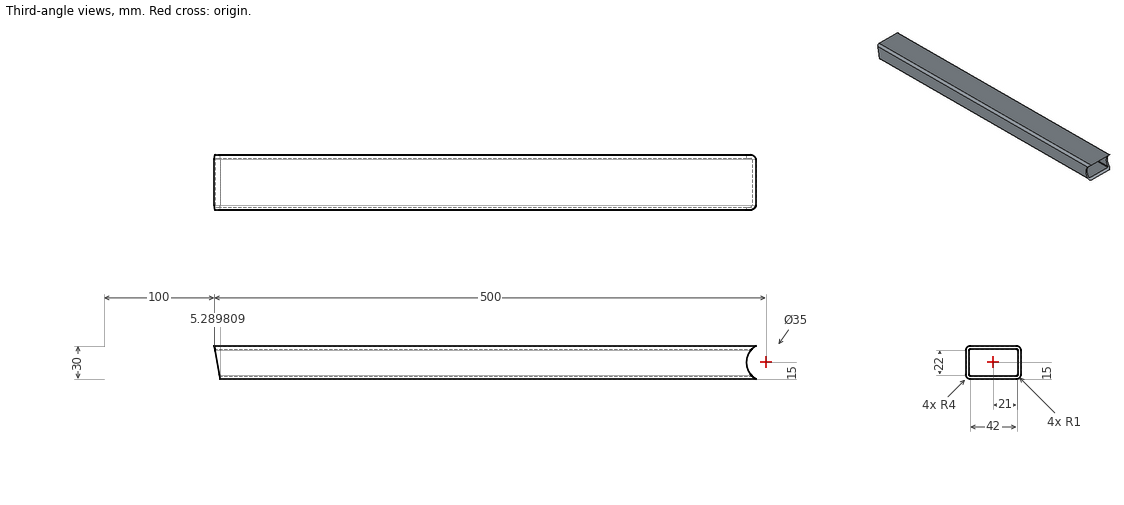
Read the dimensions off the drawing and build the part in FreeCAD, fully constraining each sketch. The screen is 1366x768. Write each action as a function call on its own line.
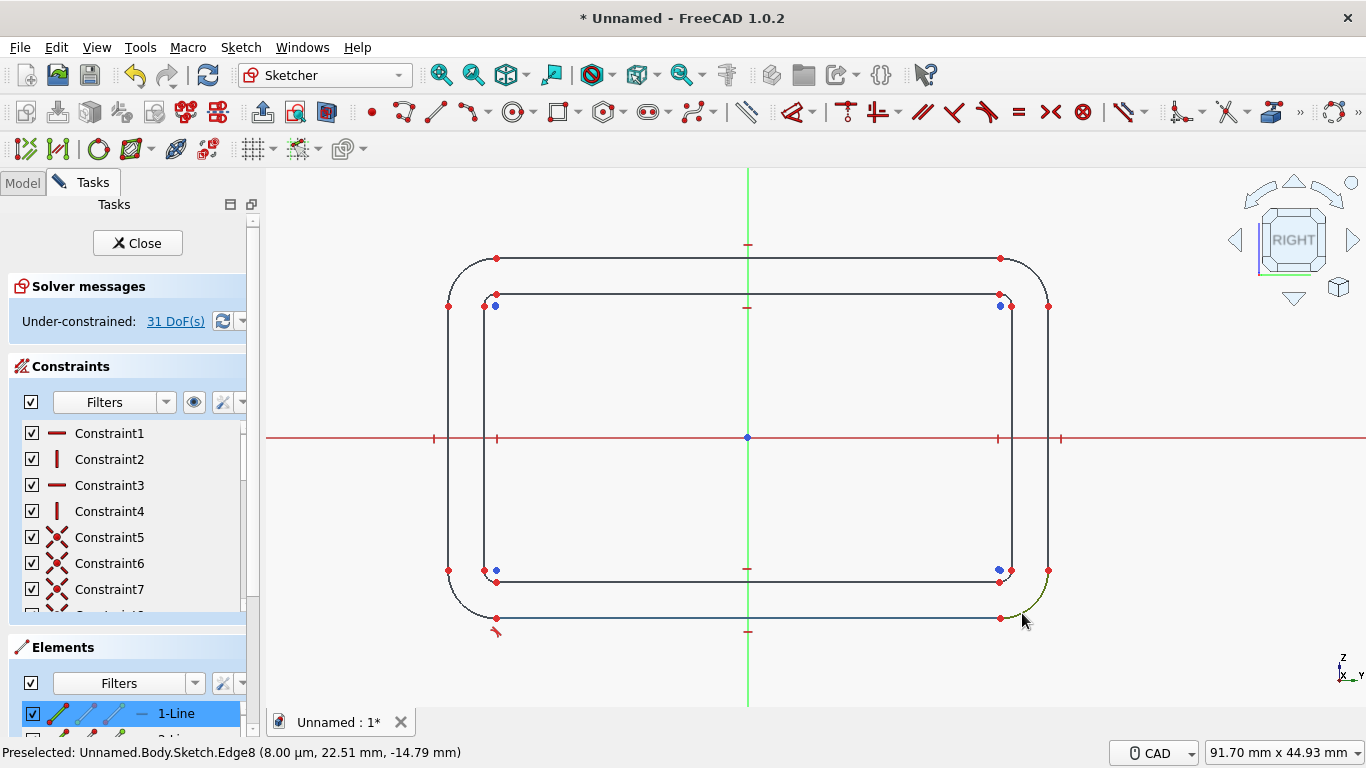
click(988, 112)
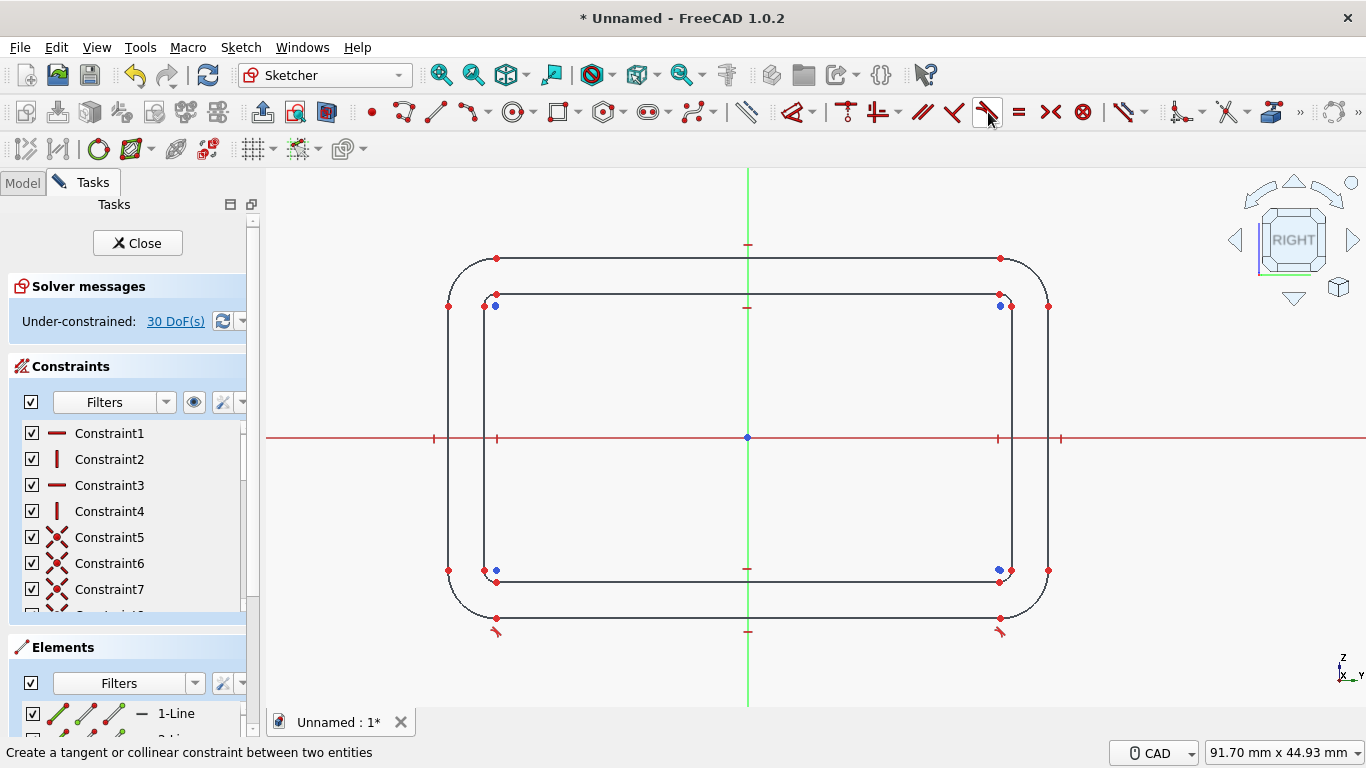
click(448, 491)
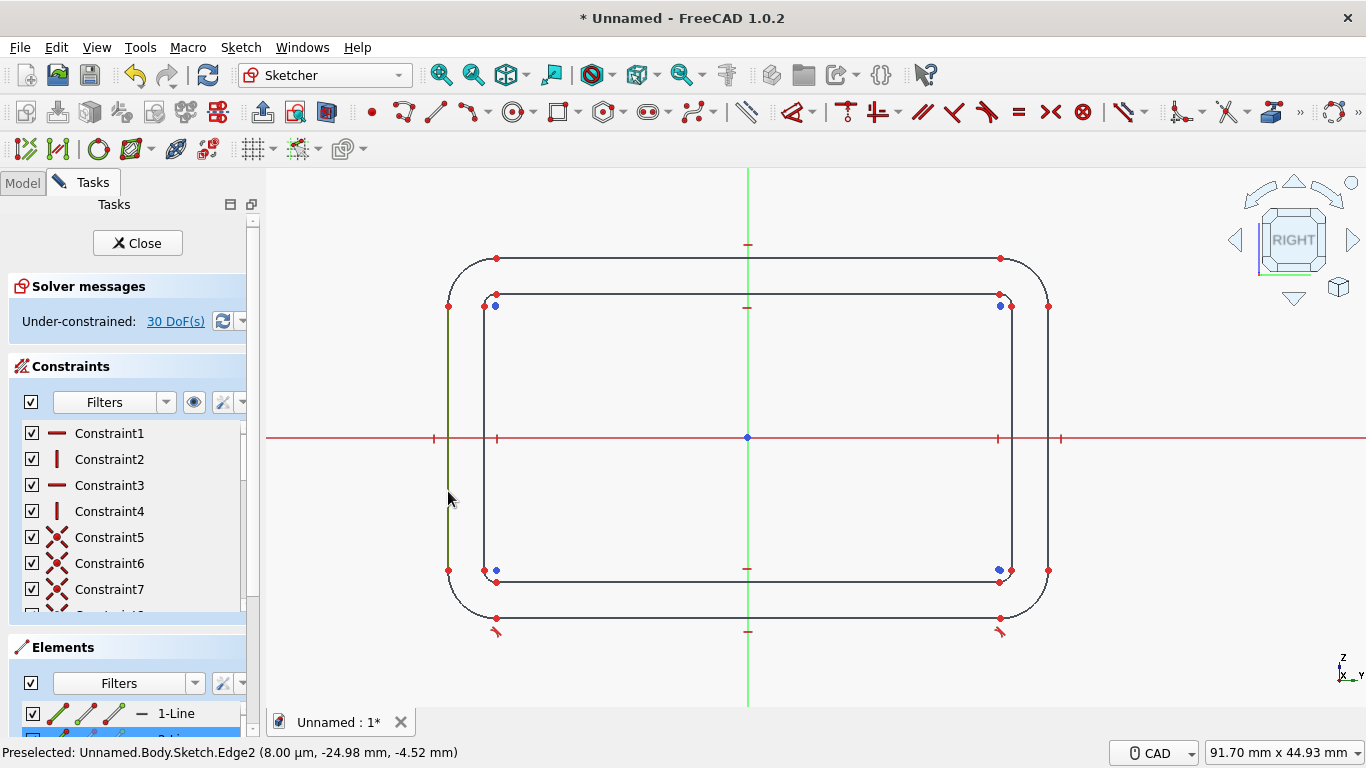
click(453, 592)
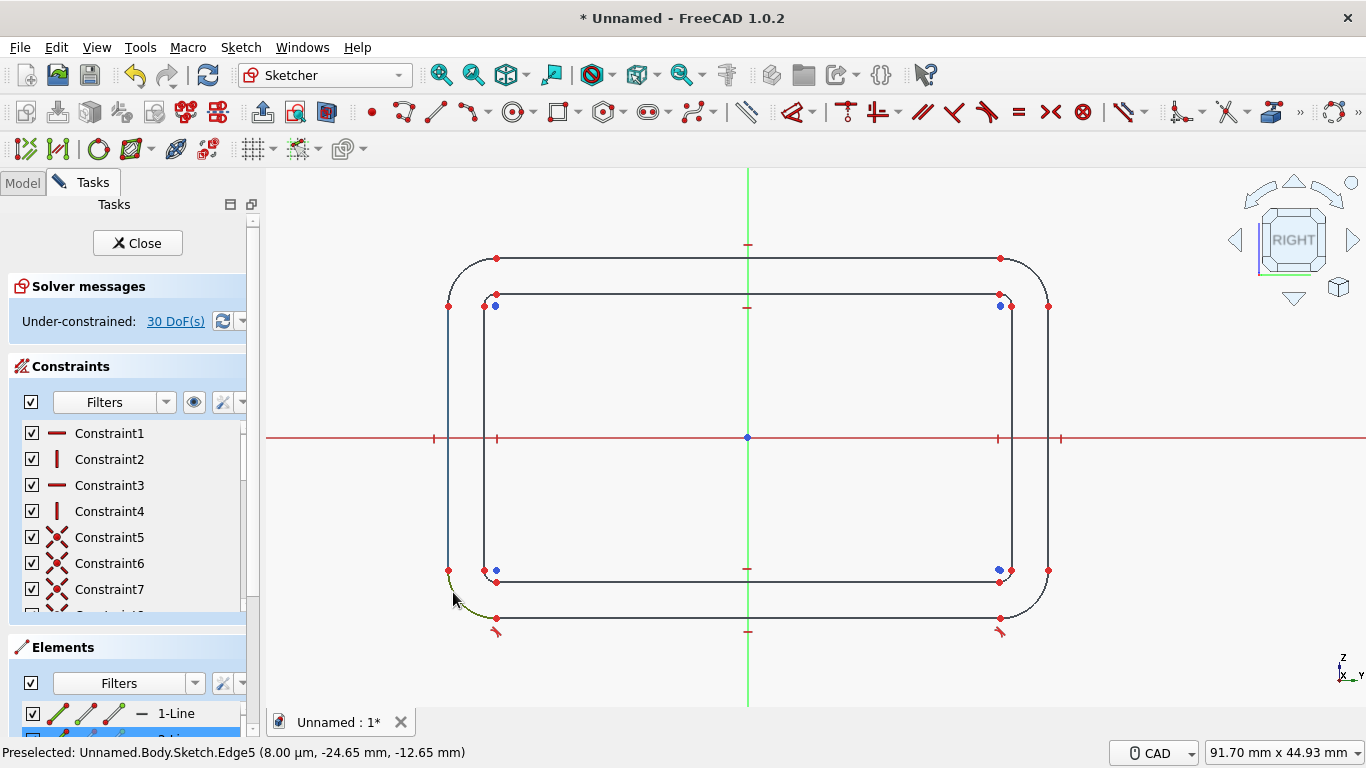
click(988, 112)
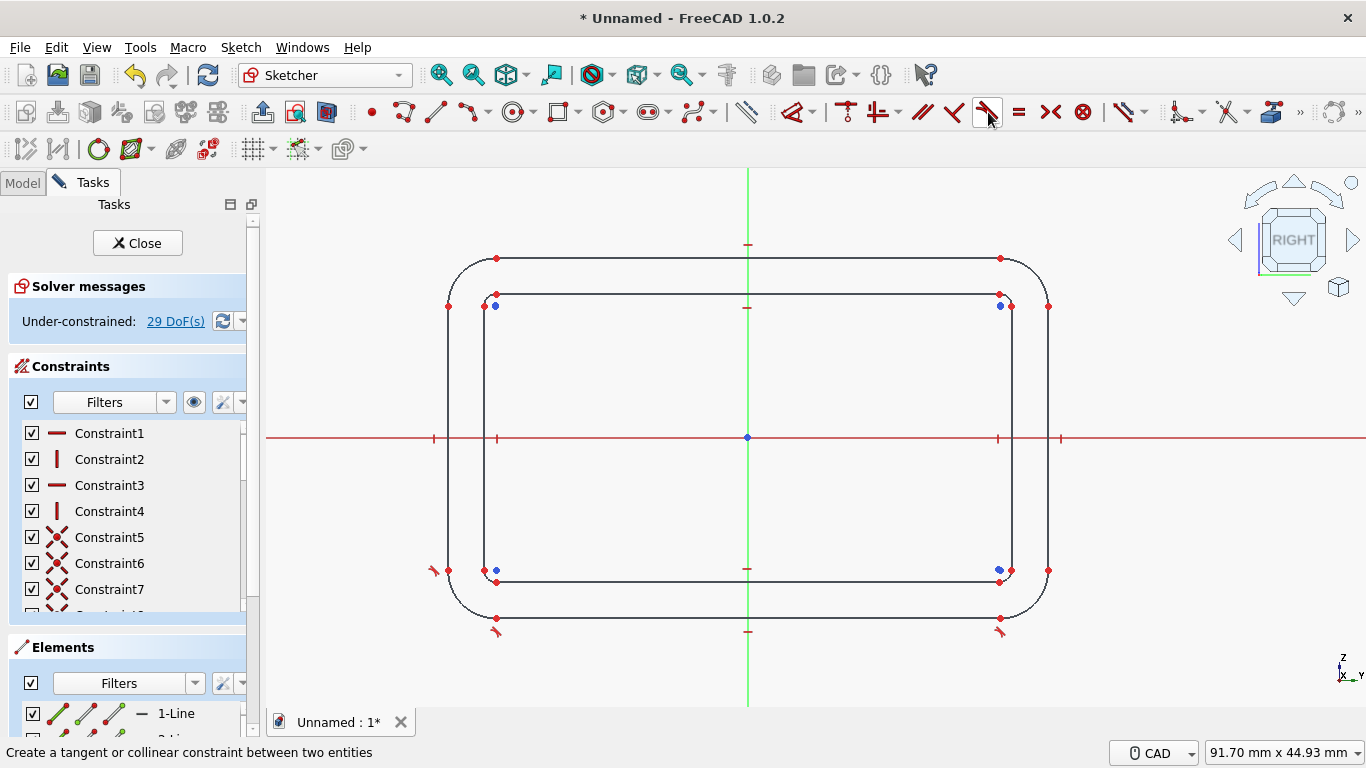
click(448, 491)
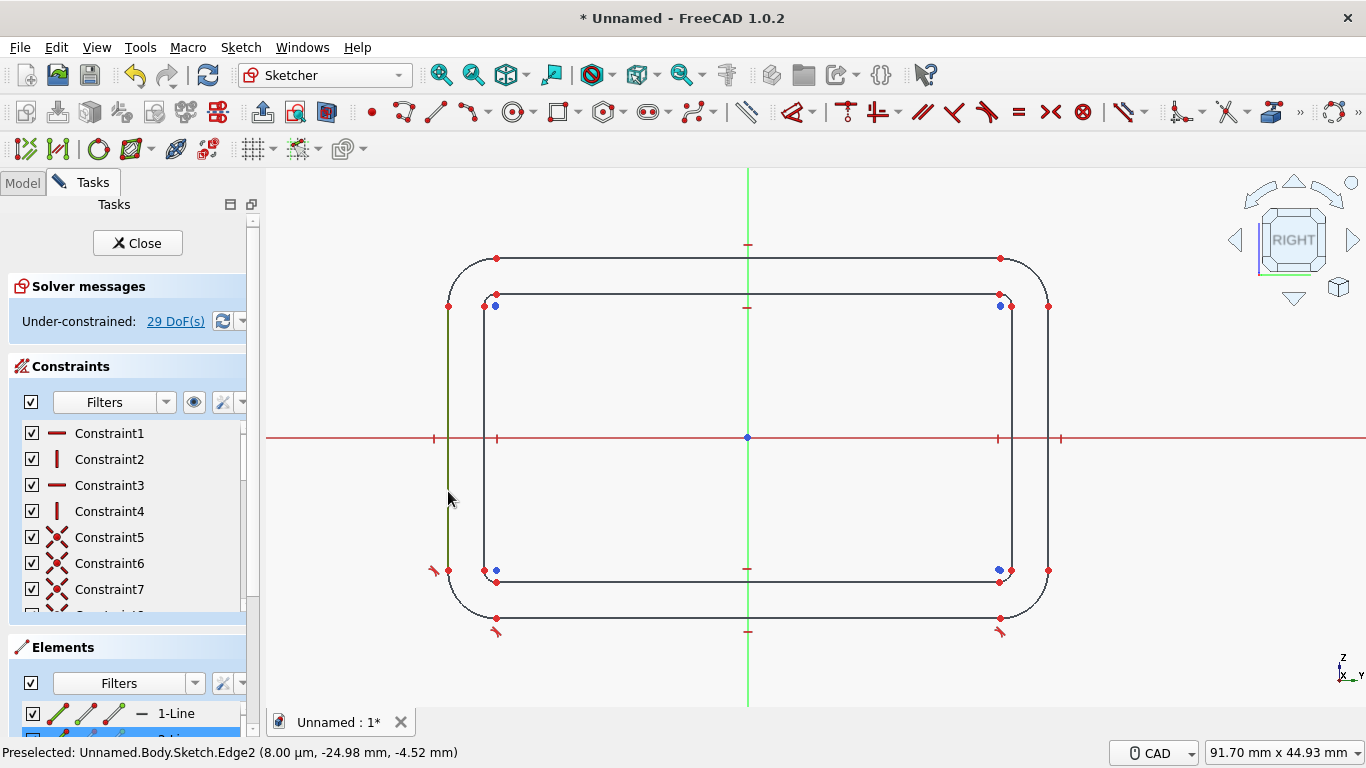
click(474, 264)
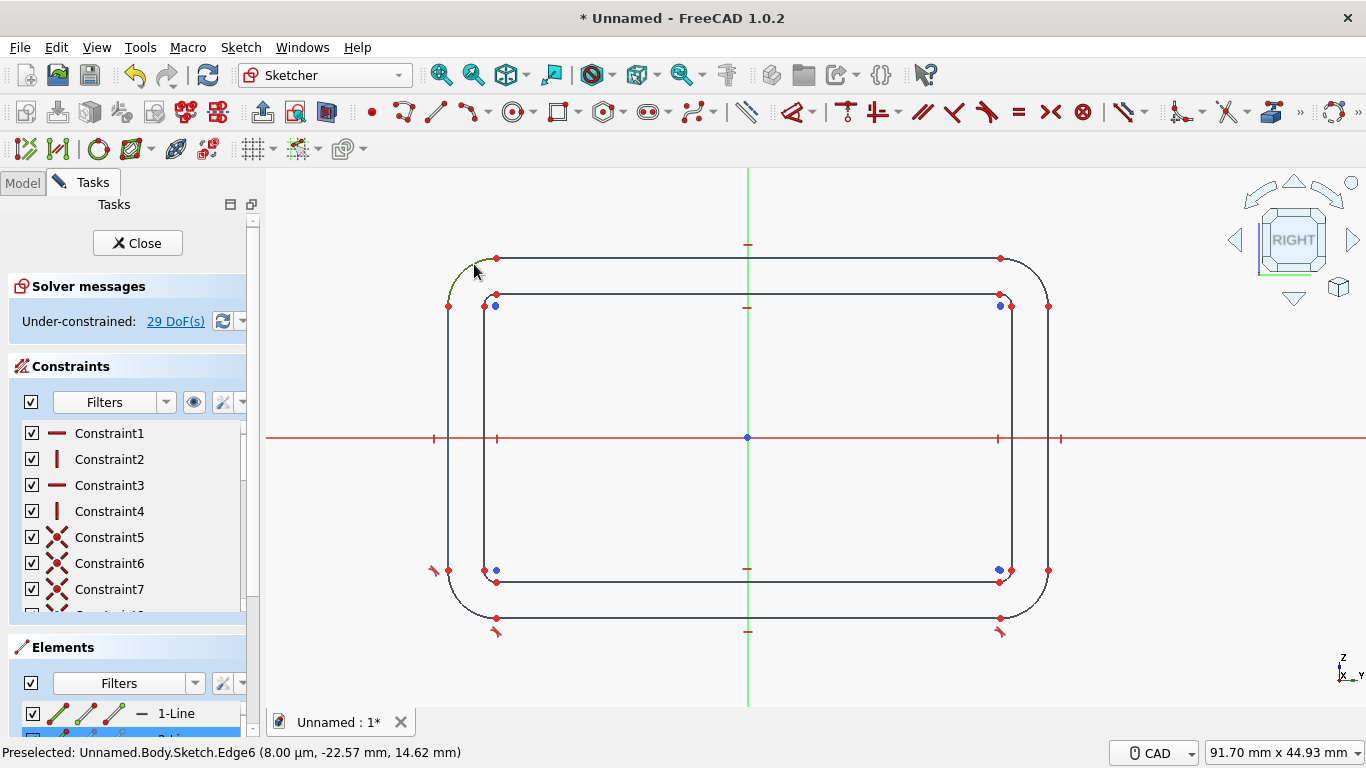
key(t)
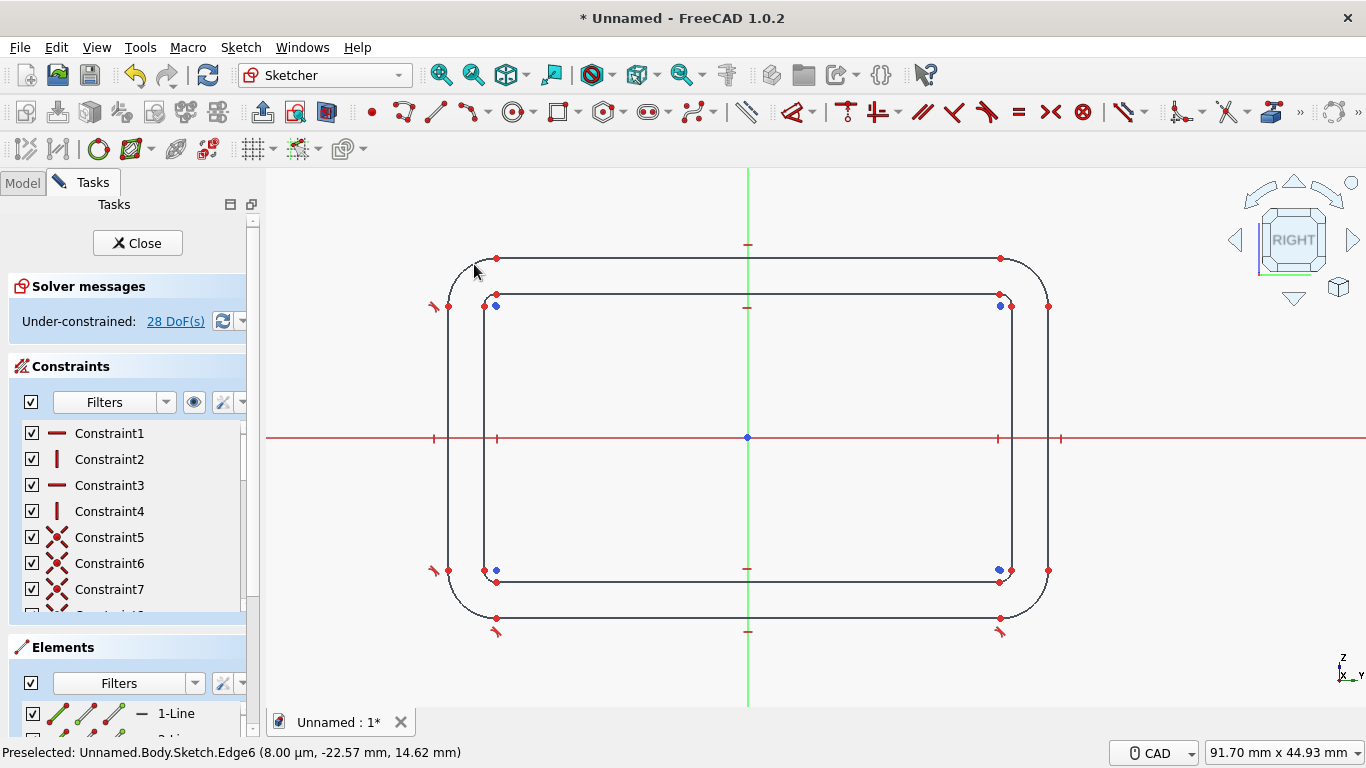
click(647, 258)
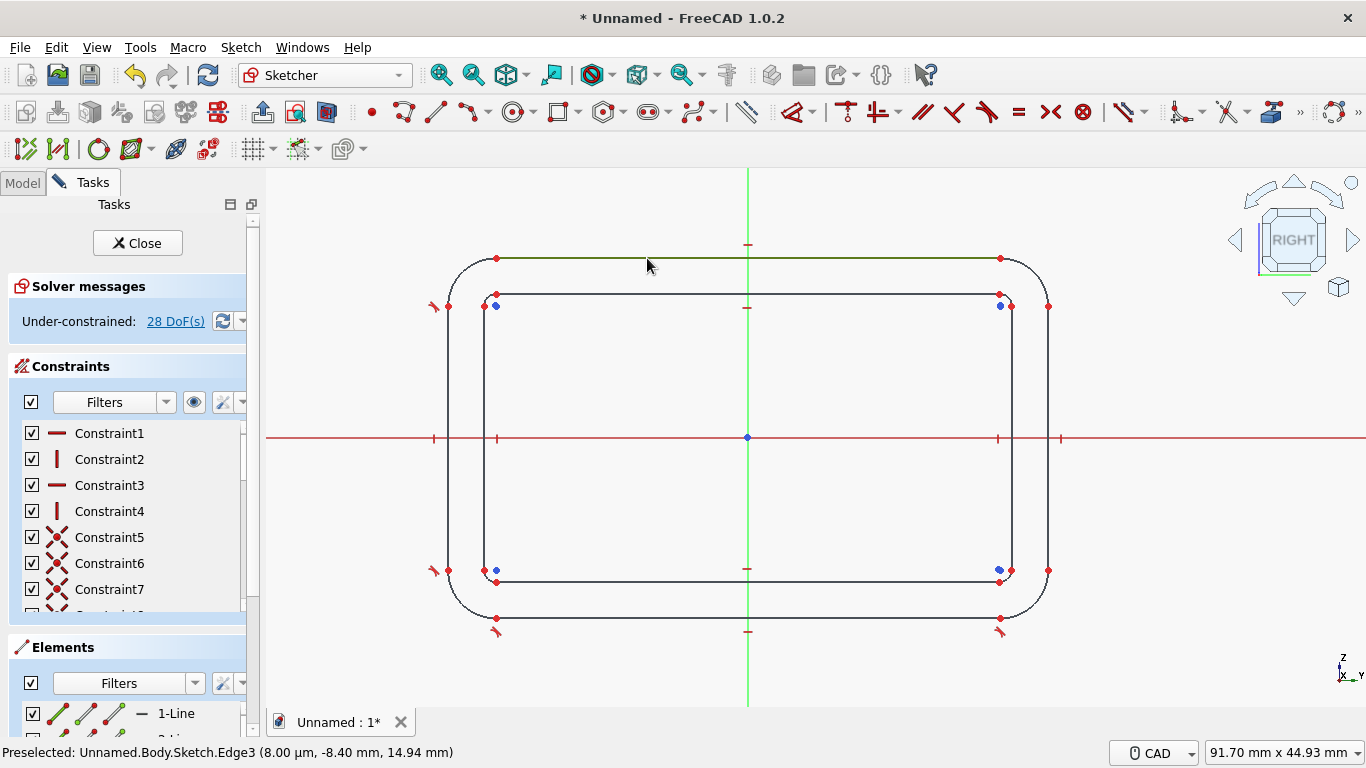
click(474, 264)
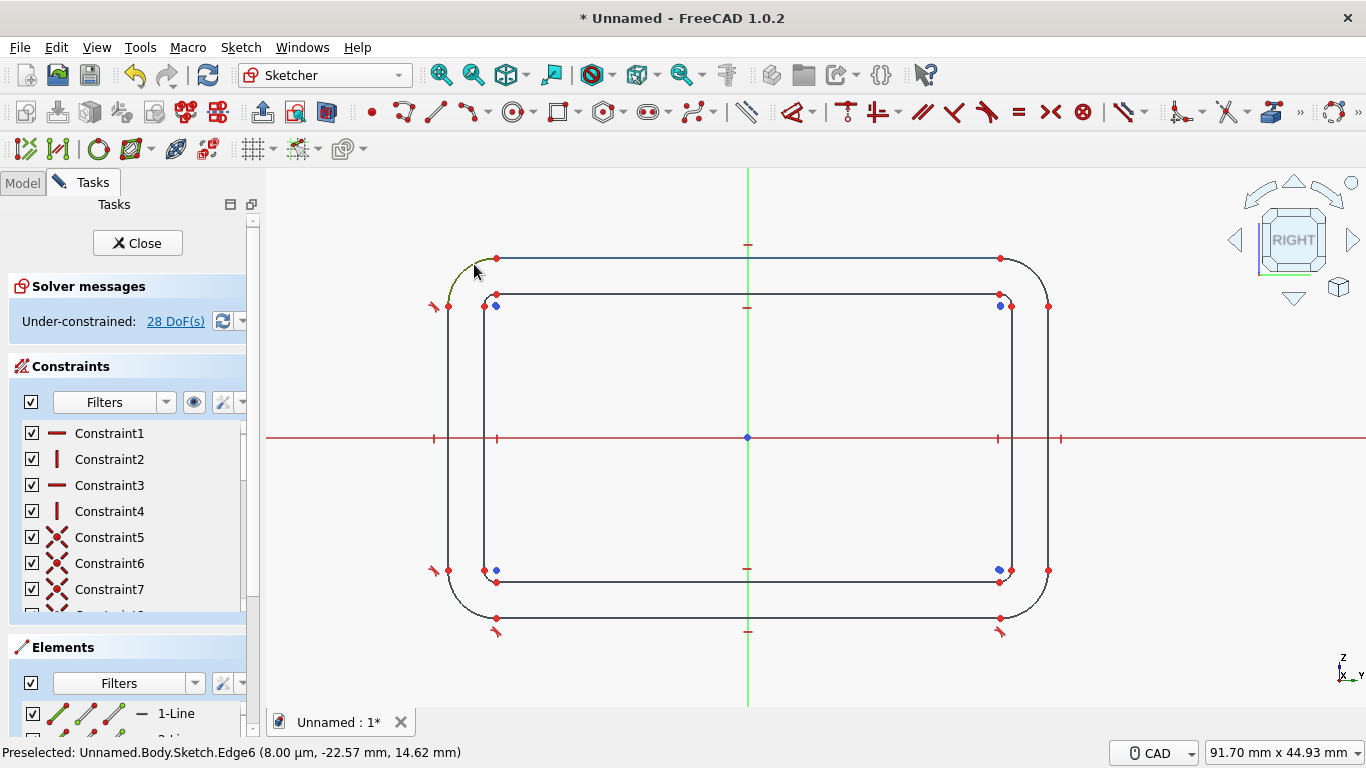
key(t)